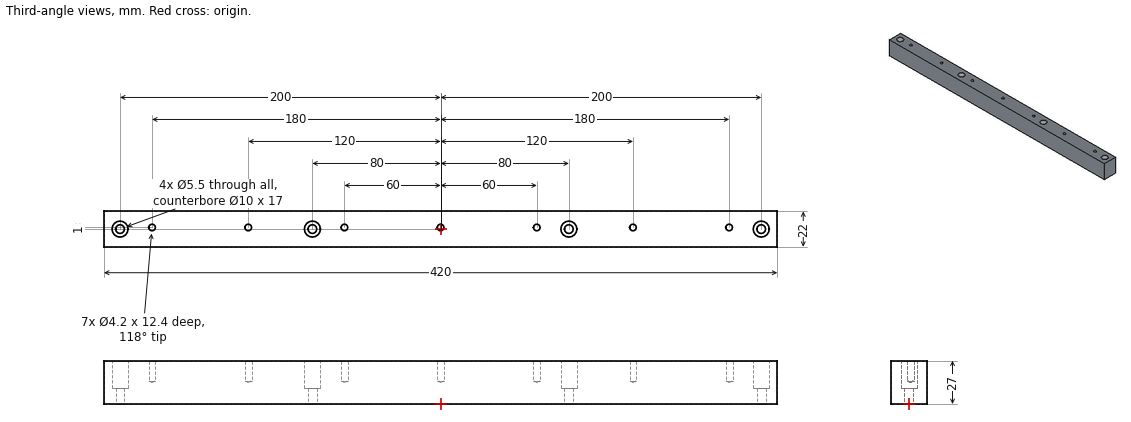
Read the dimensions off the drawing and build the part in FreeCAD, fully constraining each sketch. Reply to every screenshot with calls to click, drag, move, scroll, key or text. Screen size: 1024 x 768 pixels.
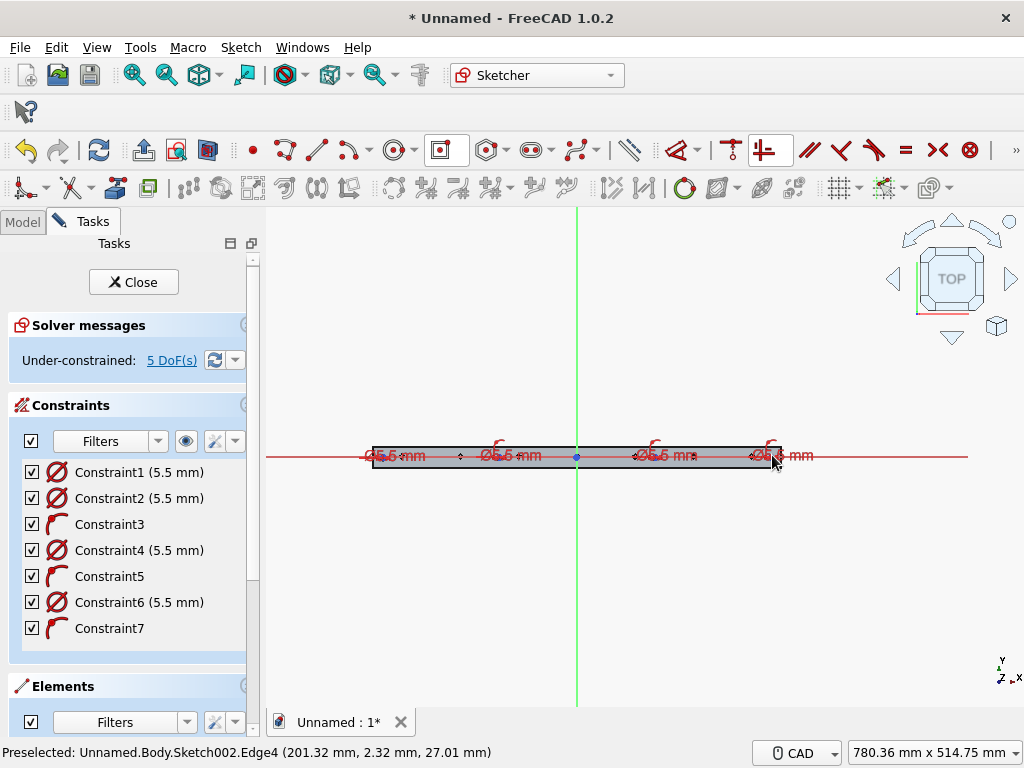
click(383, 458)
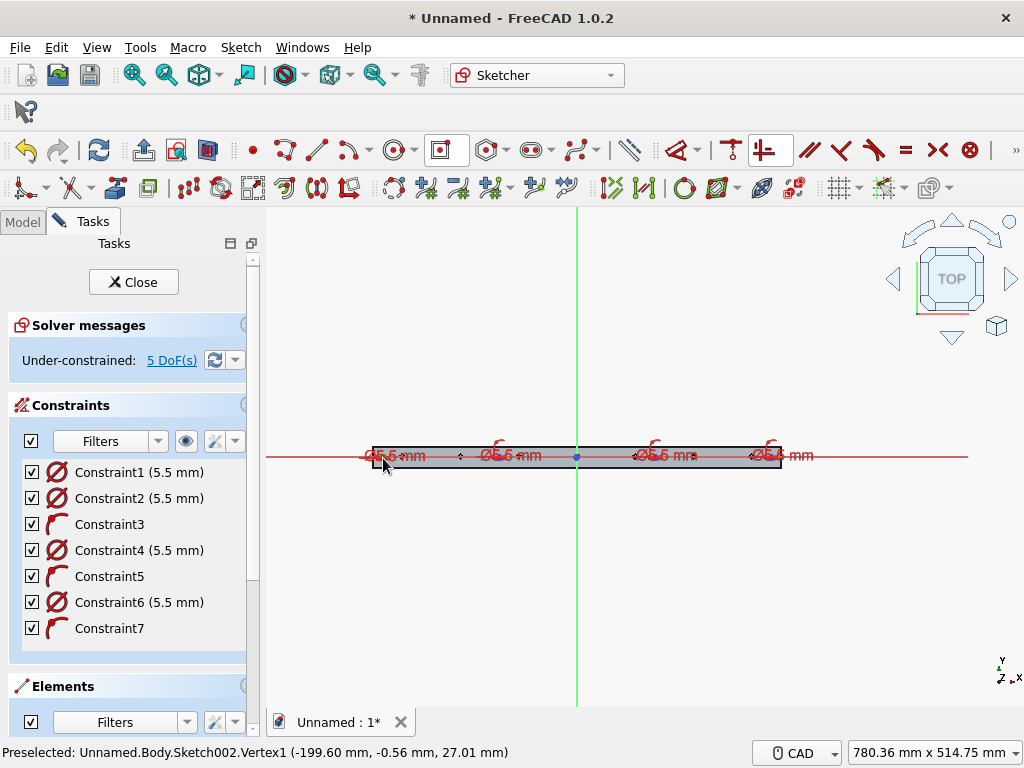
click(334, 457)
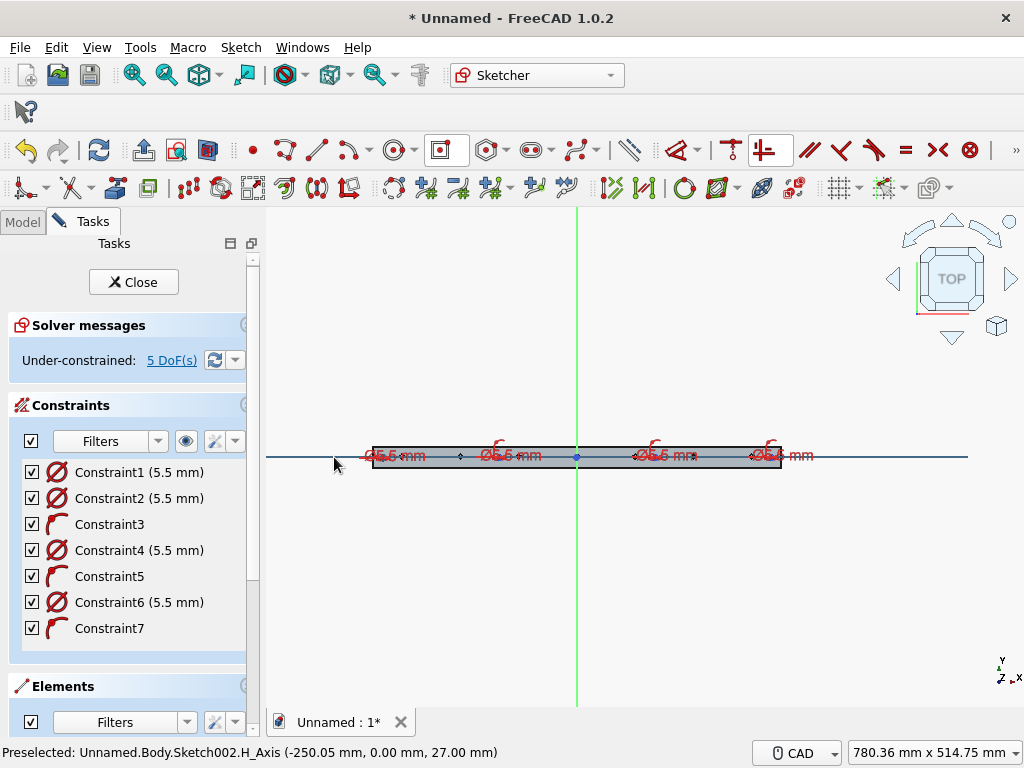
key(c)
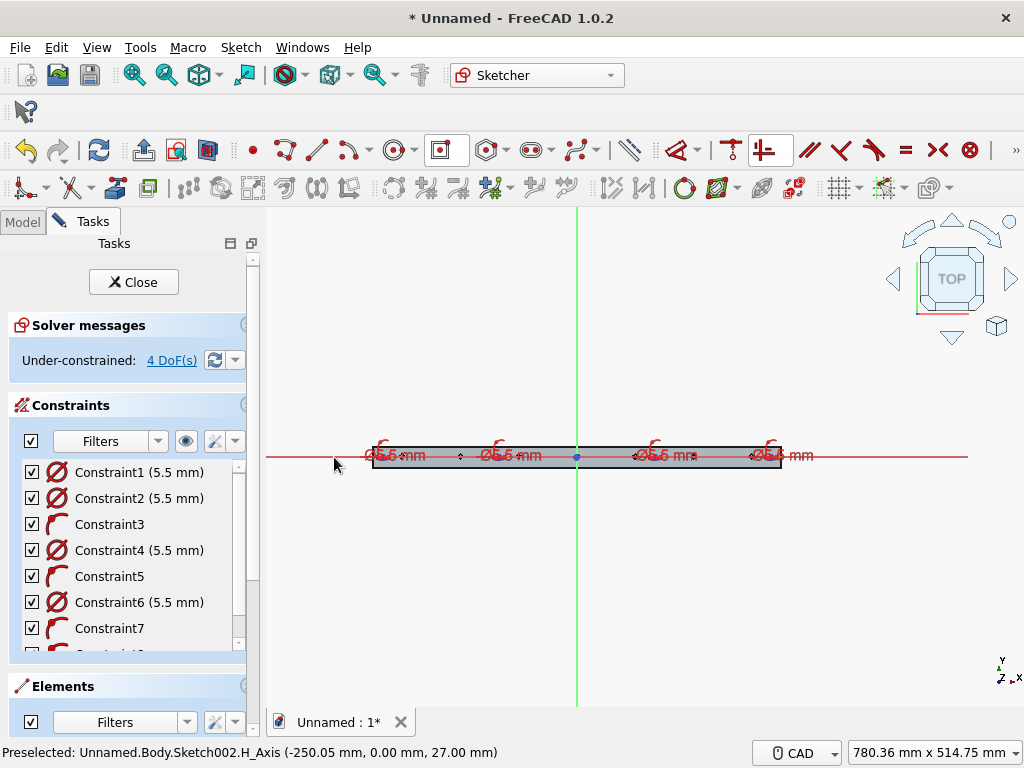
click(676, 150)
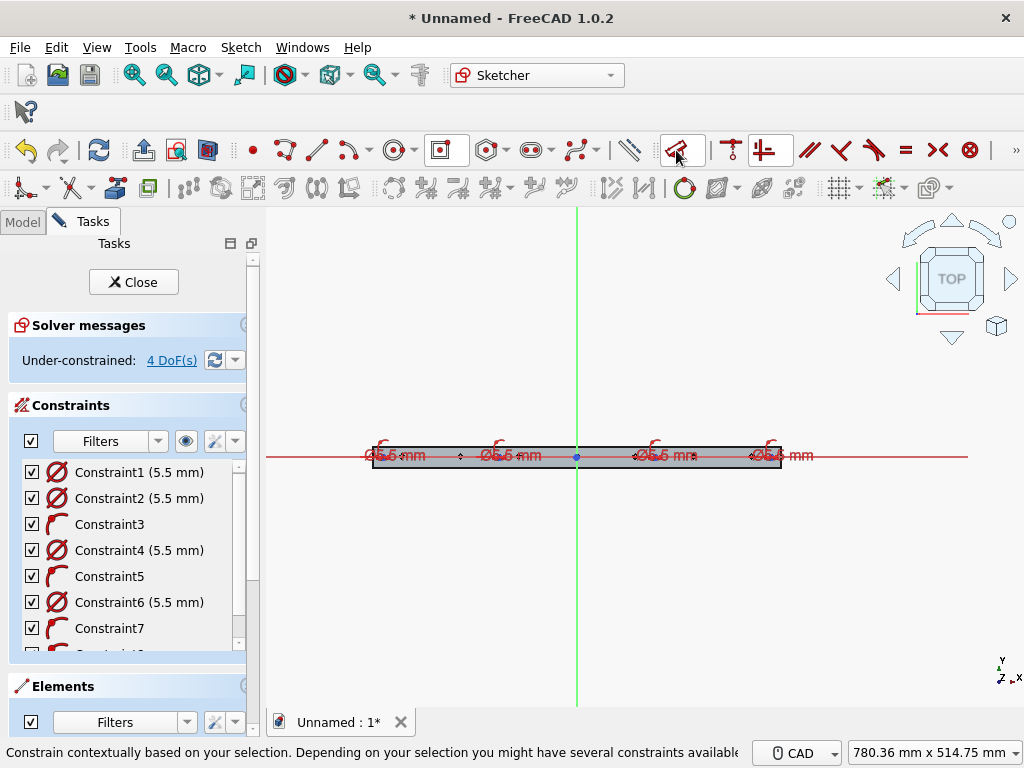
click(499, 457)
click(538, 491)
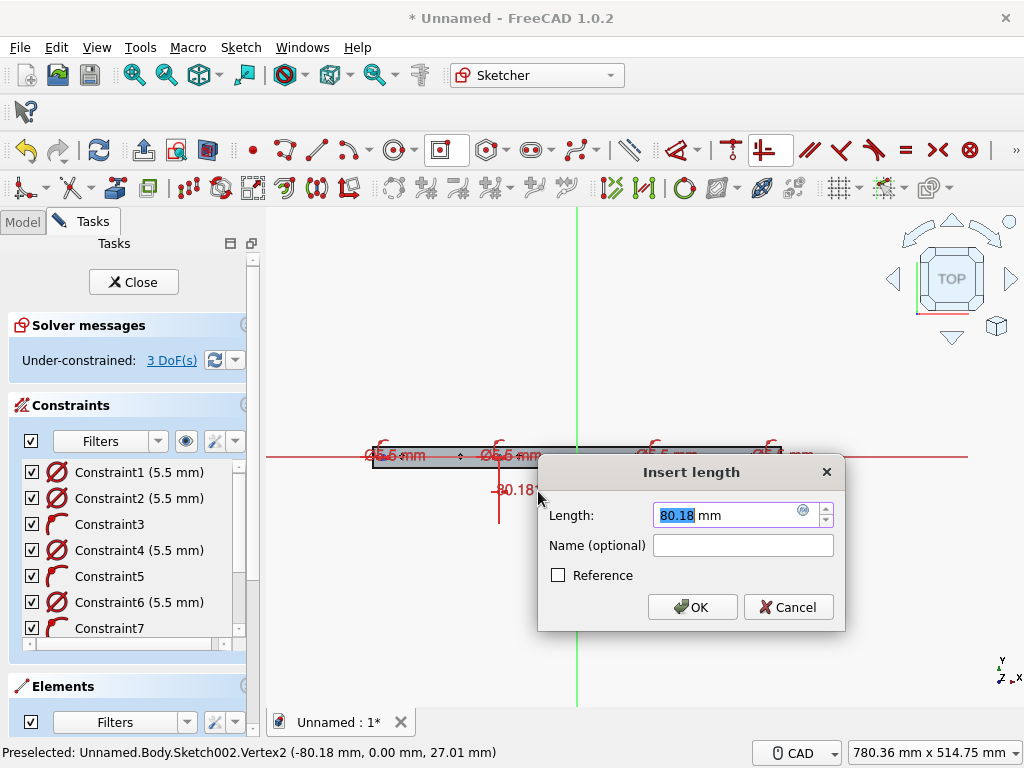
text(80)
key(Return)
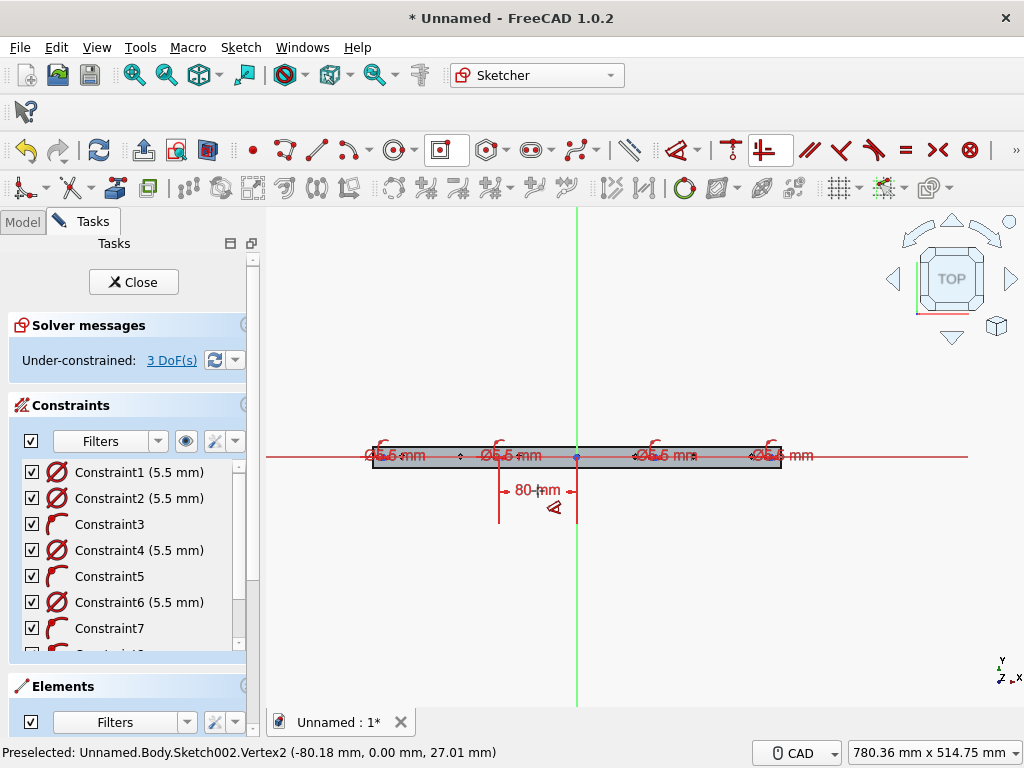
click(655, 457)
click(616, 491)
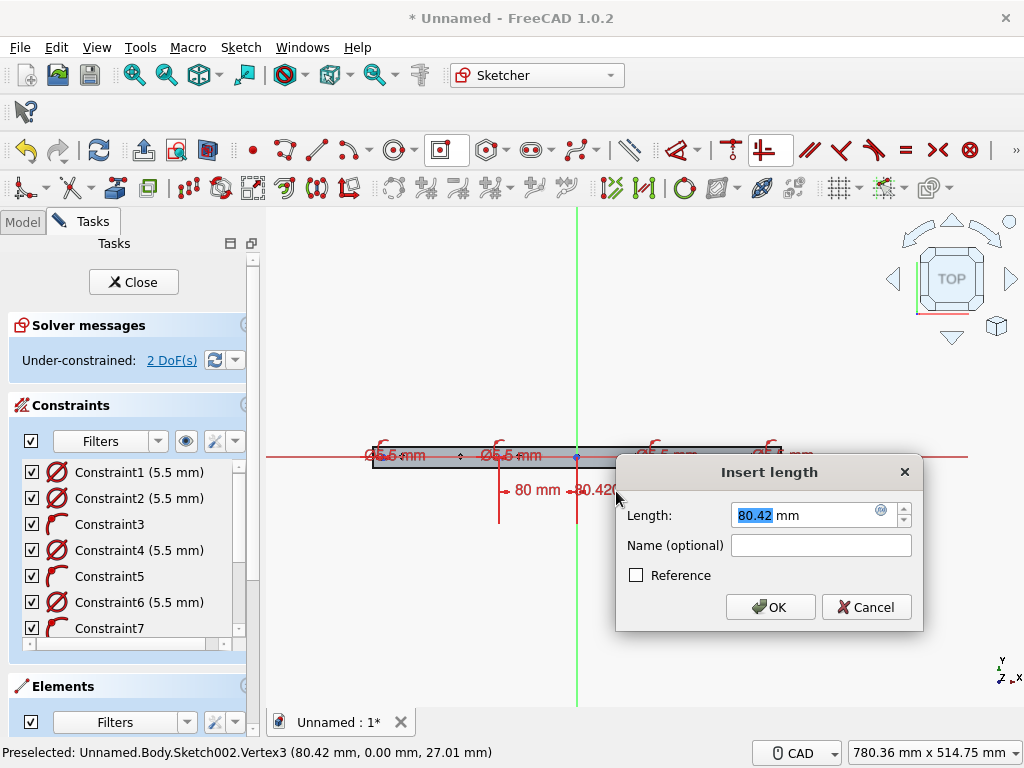
text(80)
key(Return)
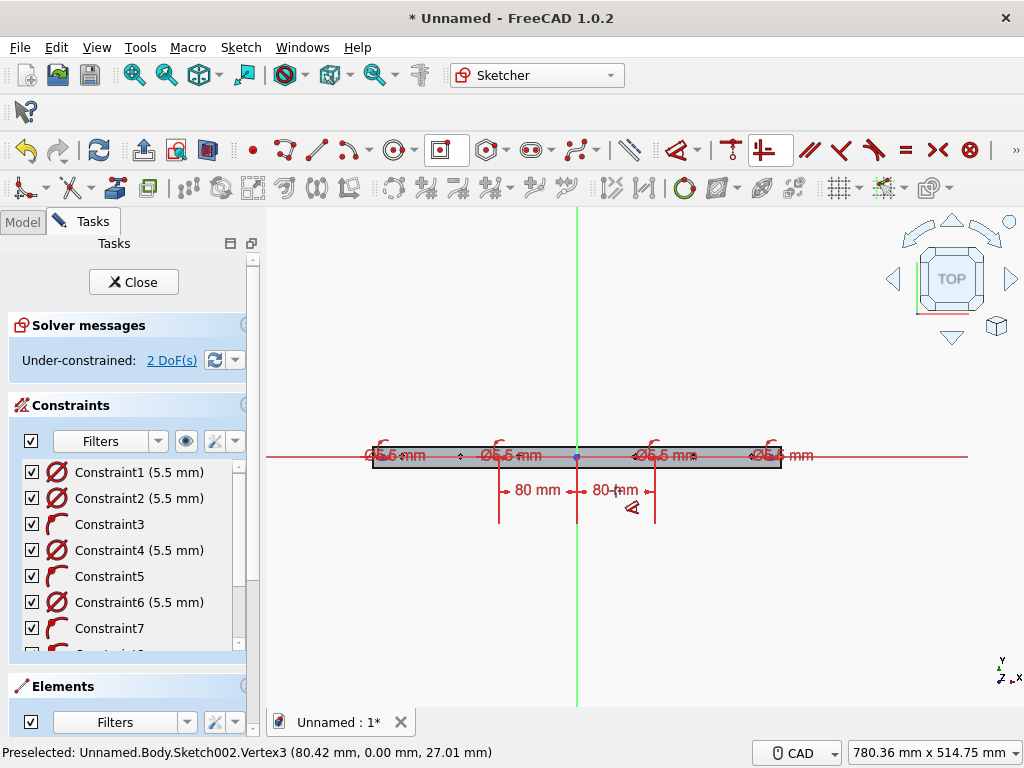
click(383, 457)
click(435, 491)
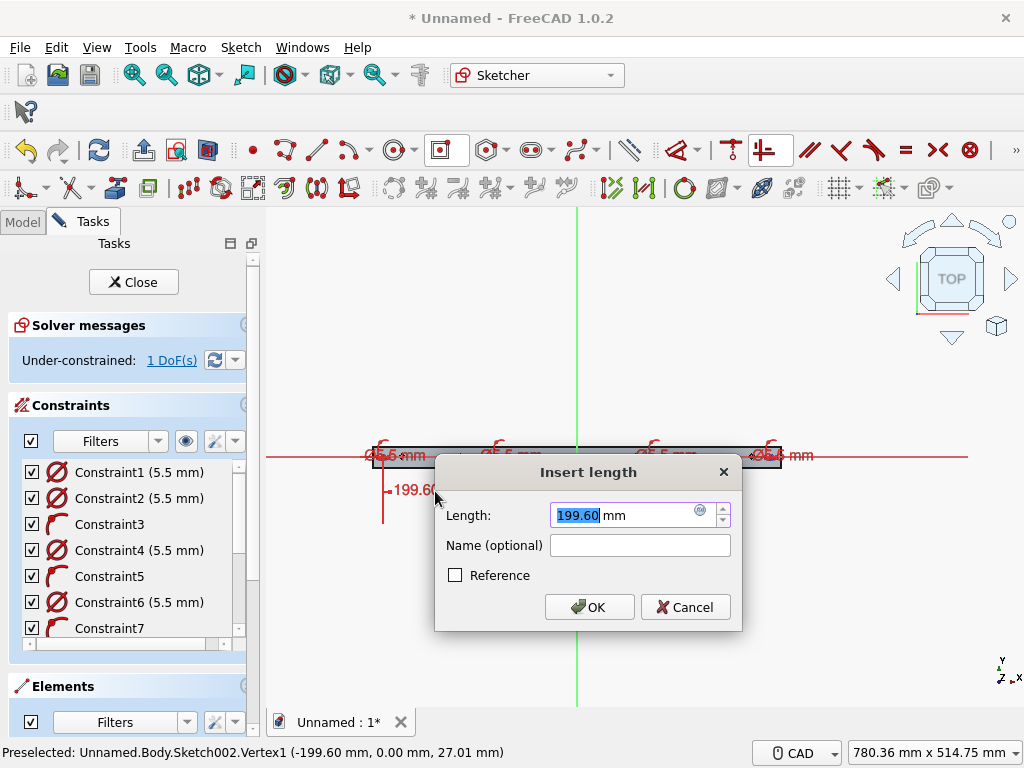
text(200)
key(Return)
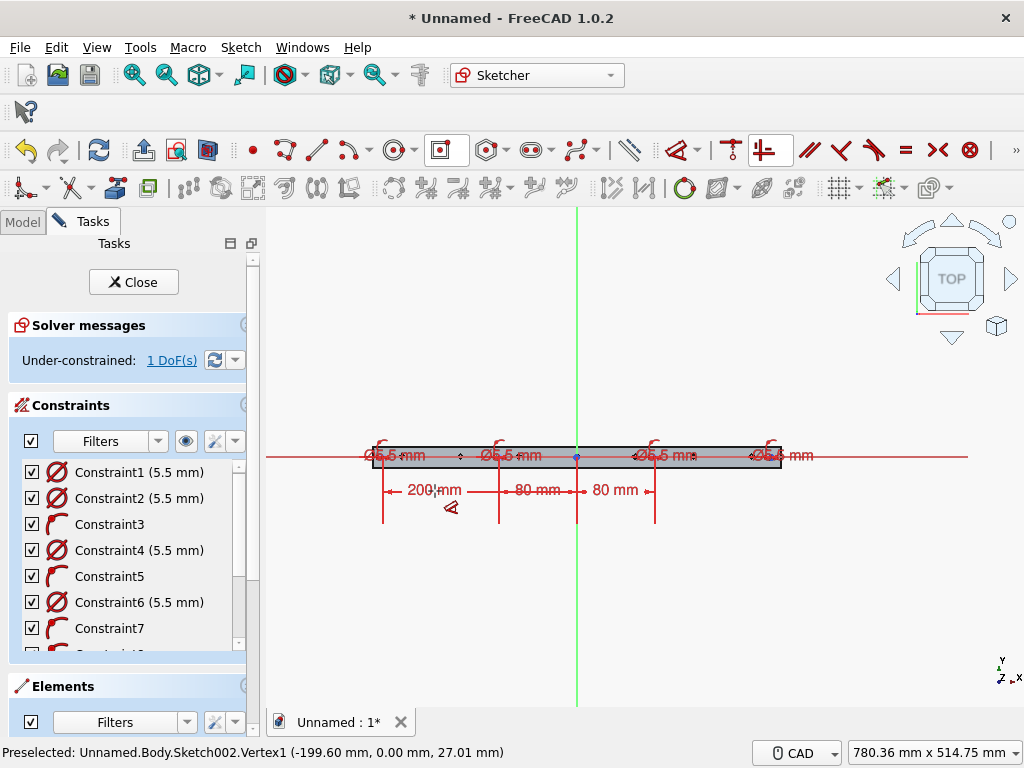
click(771, 457)
click(719, 491)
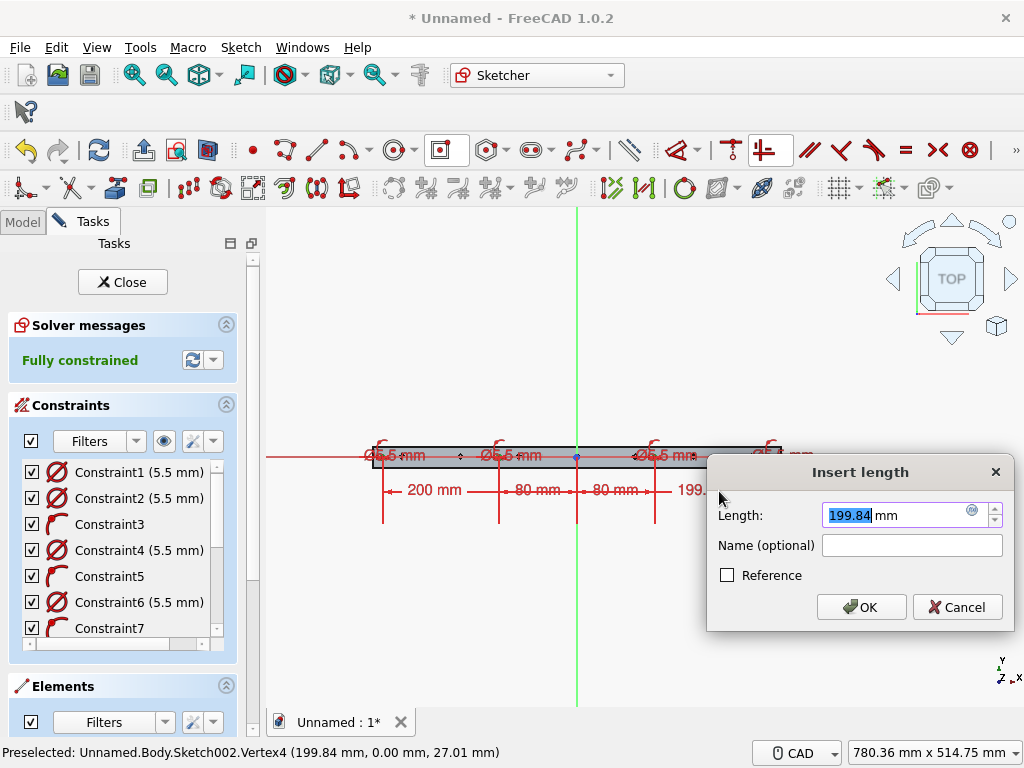
text(200)
key(Return)
key(Escape)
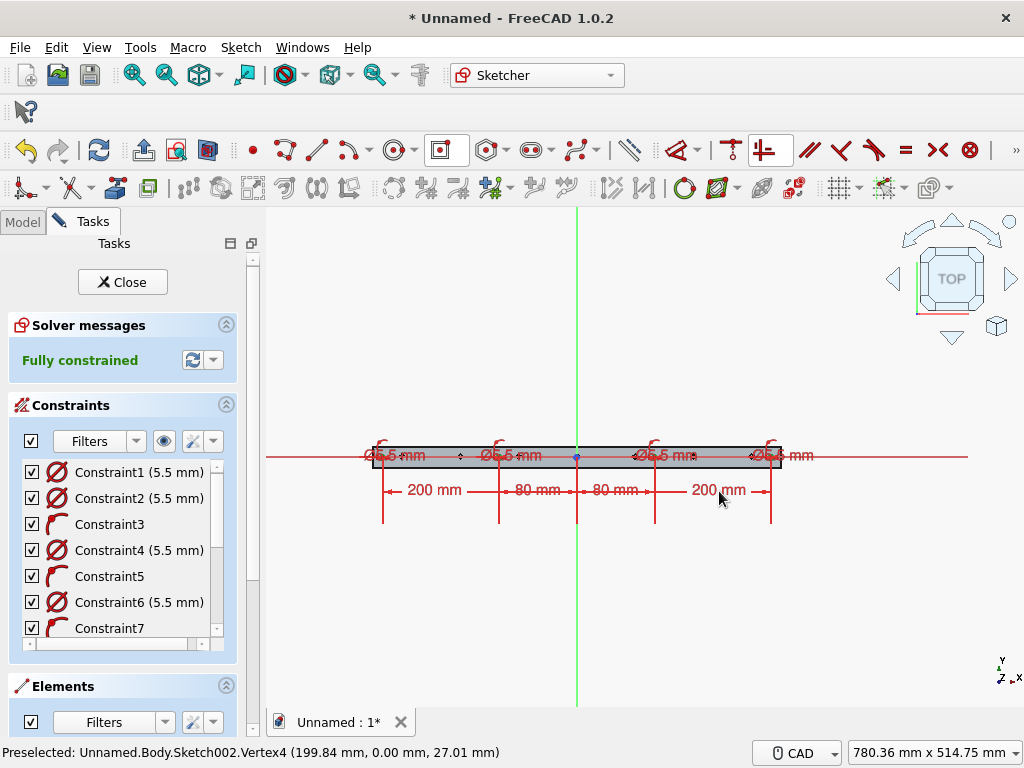
click(123, 282)